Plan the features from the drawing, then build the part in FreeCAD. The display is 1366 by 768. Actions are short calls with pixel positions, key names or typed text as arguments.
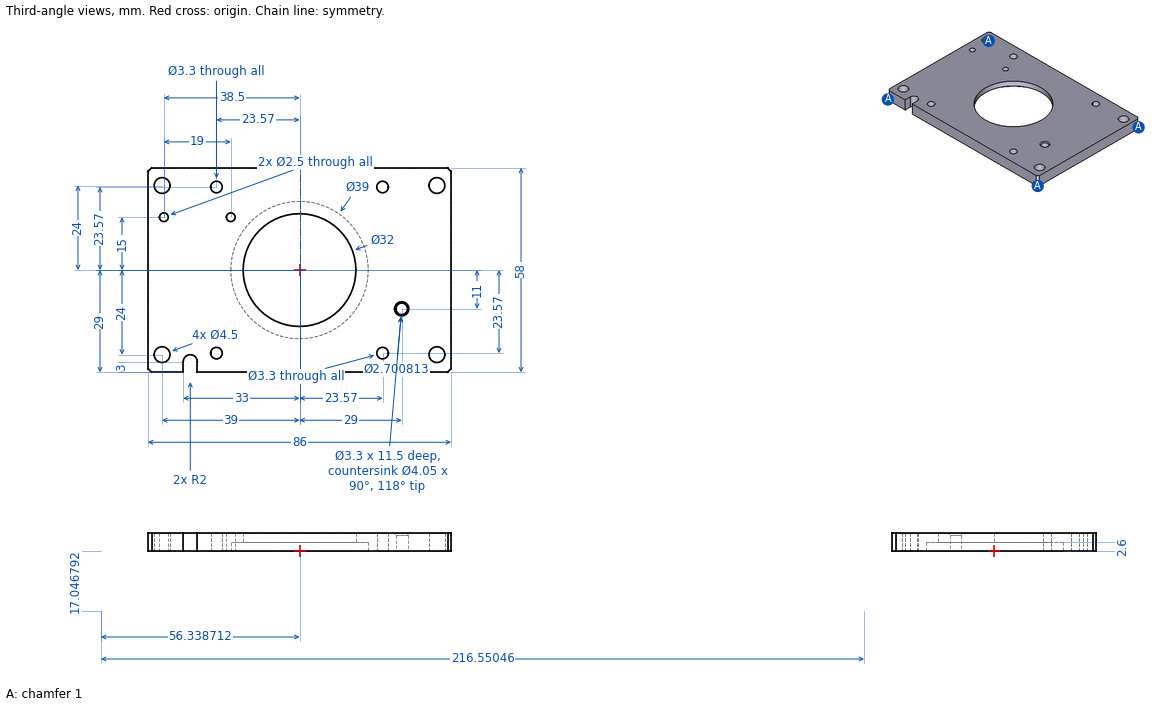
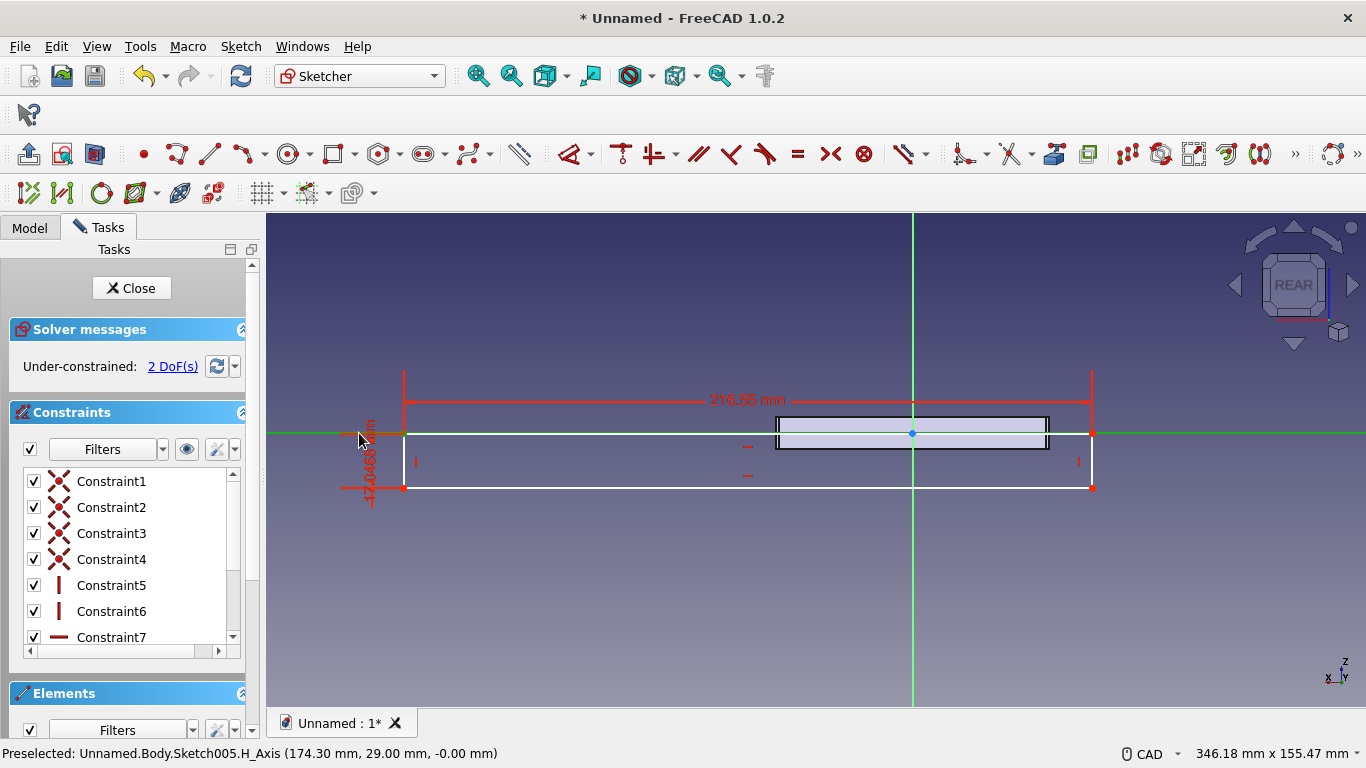
click(621, 154)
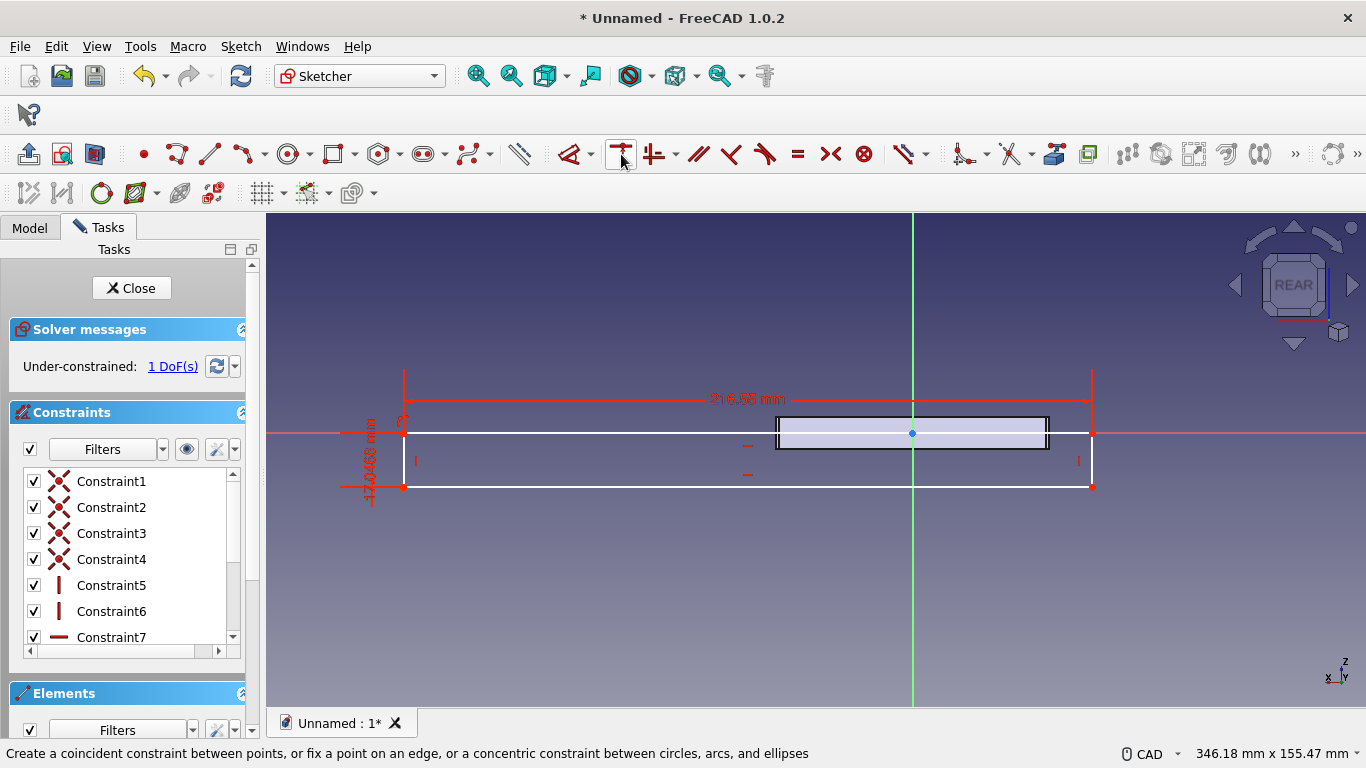
key(d)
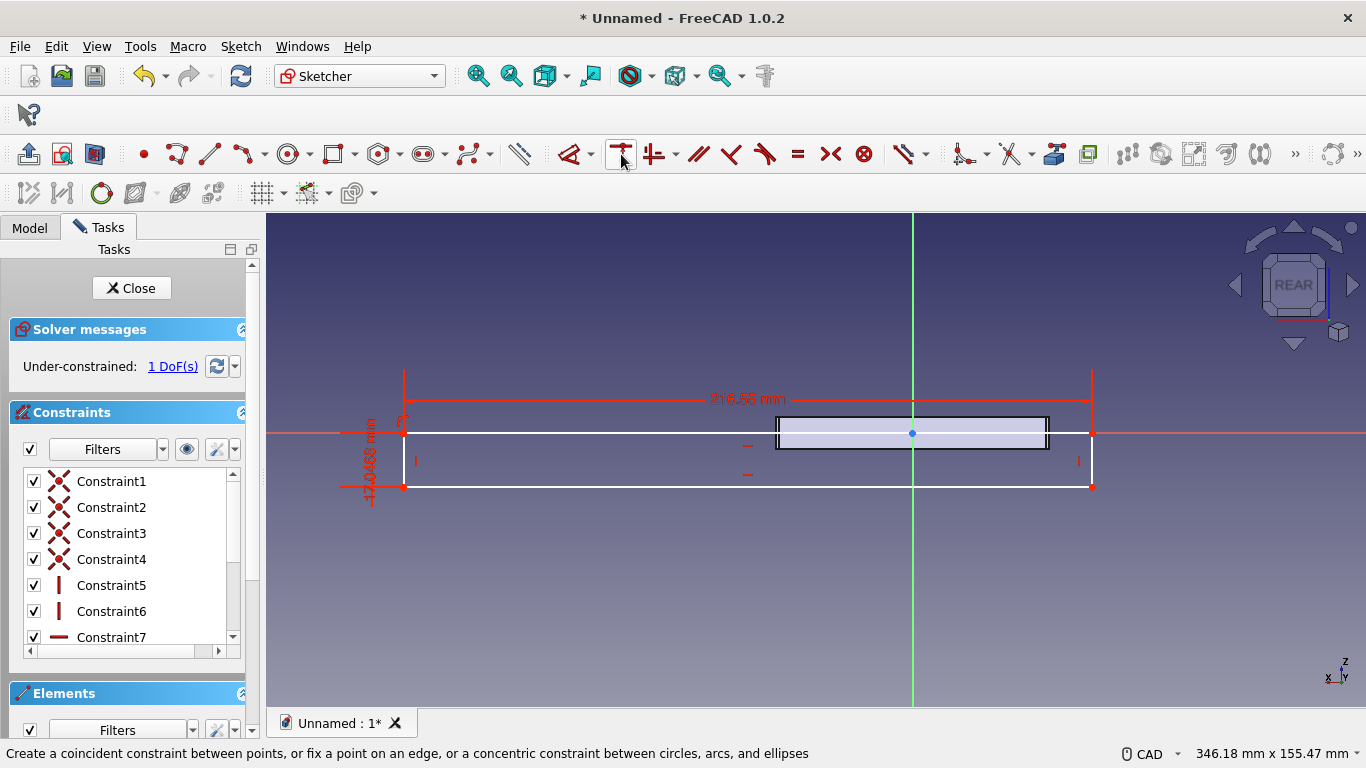
click(1092, 487)
click(1002, 399)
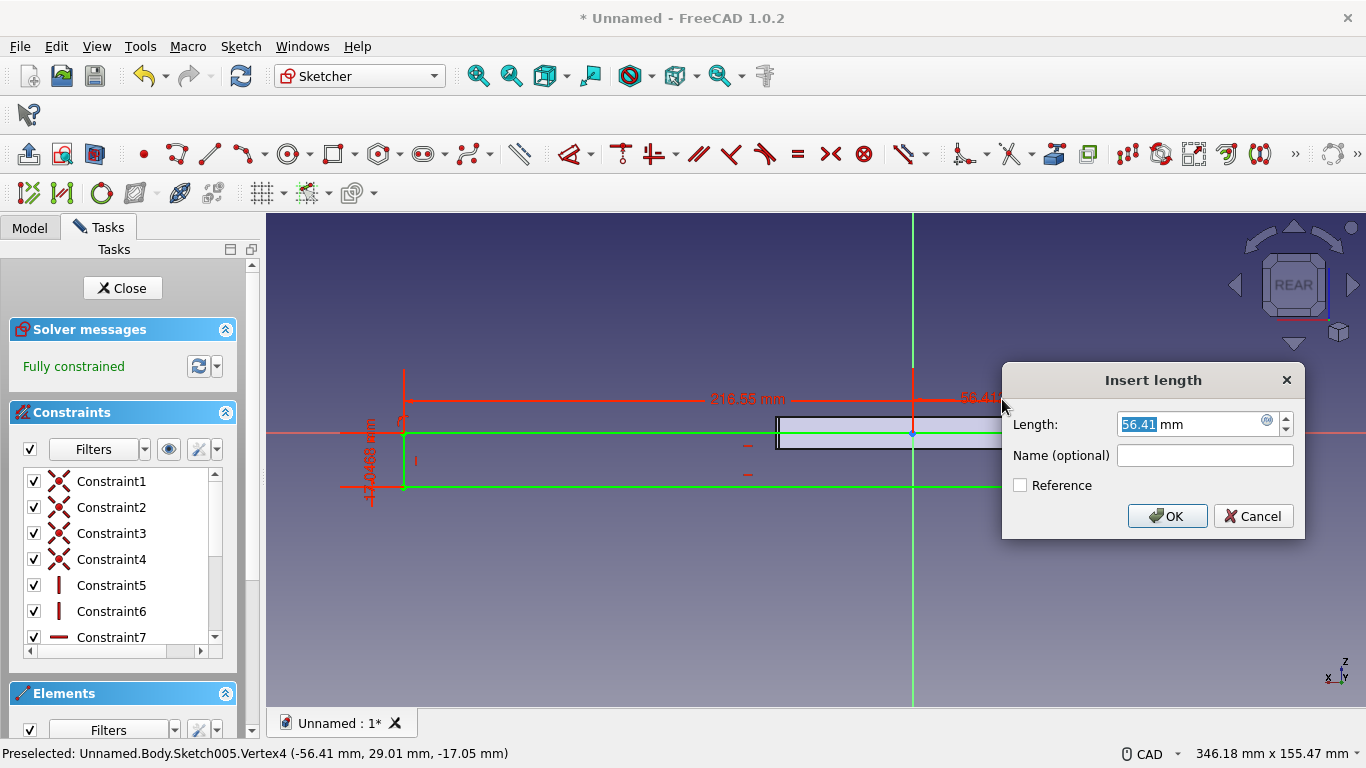
text(56.338712)
key(Return)
key(Escape)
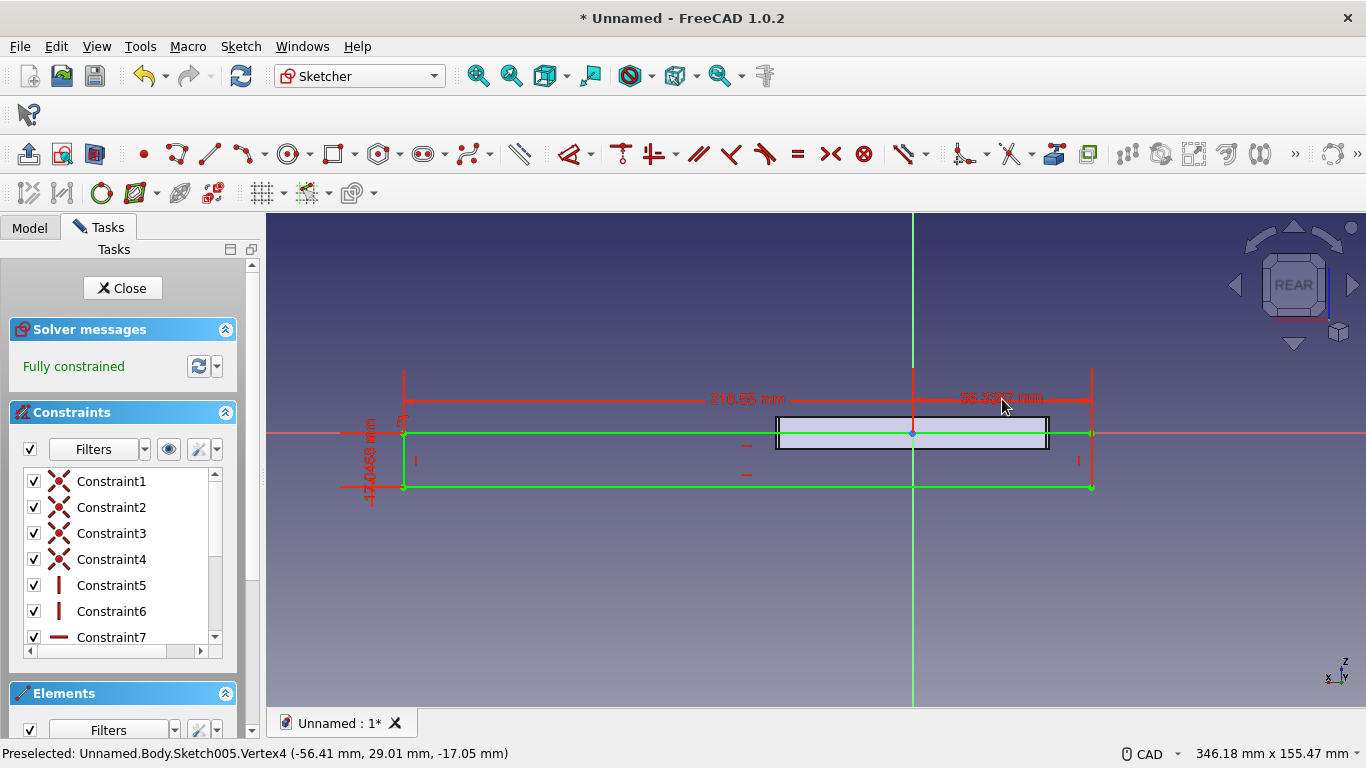
click(123, 288)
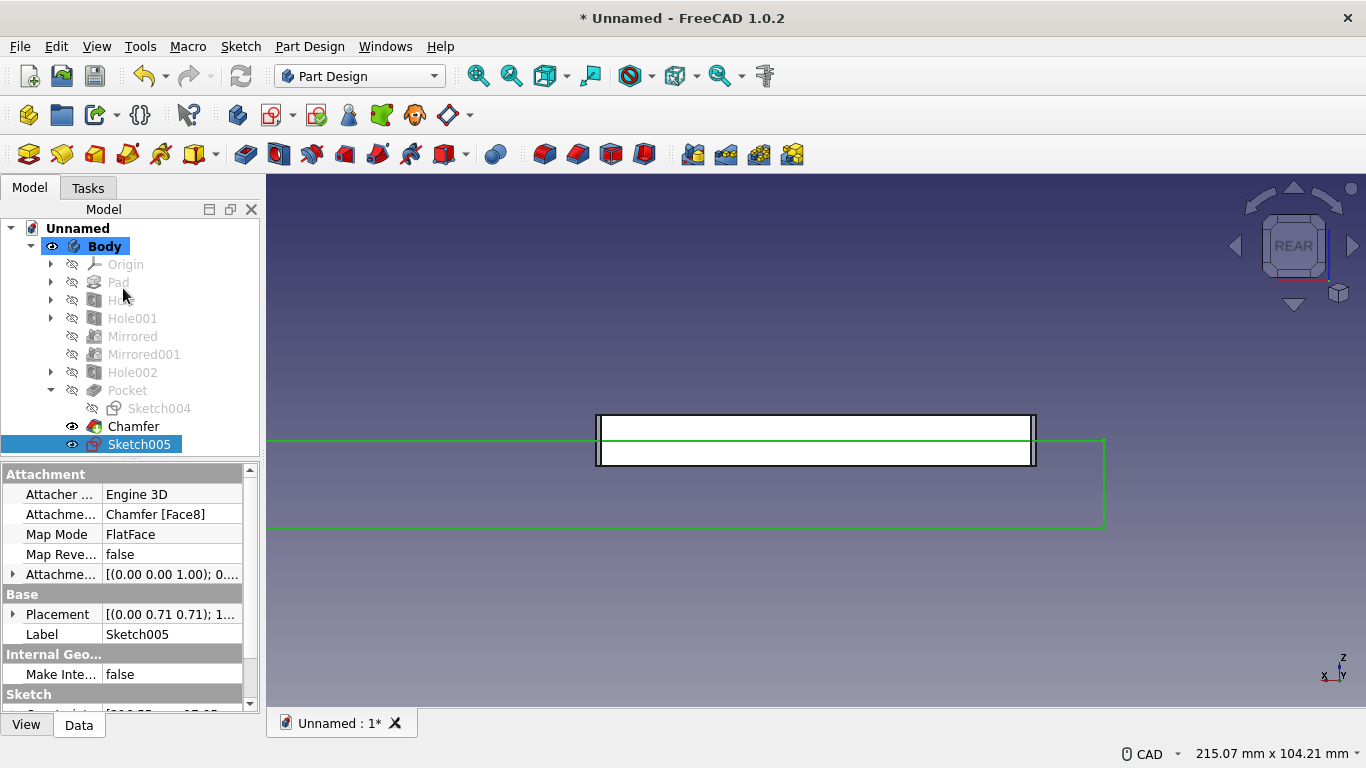
click(246, 154)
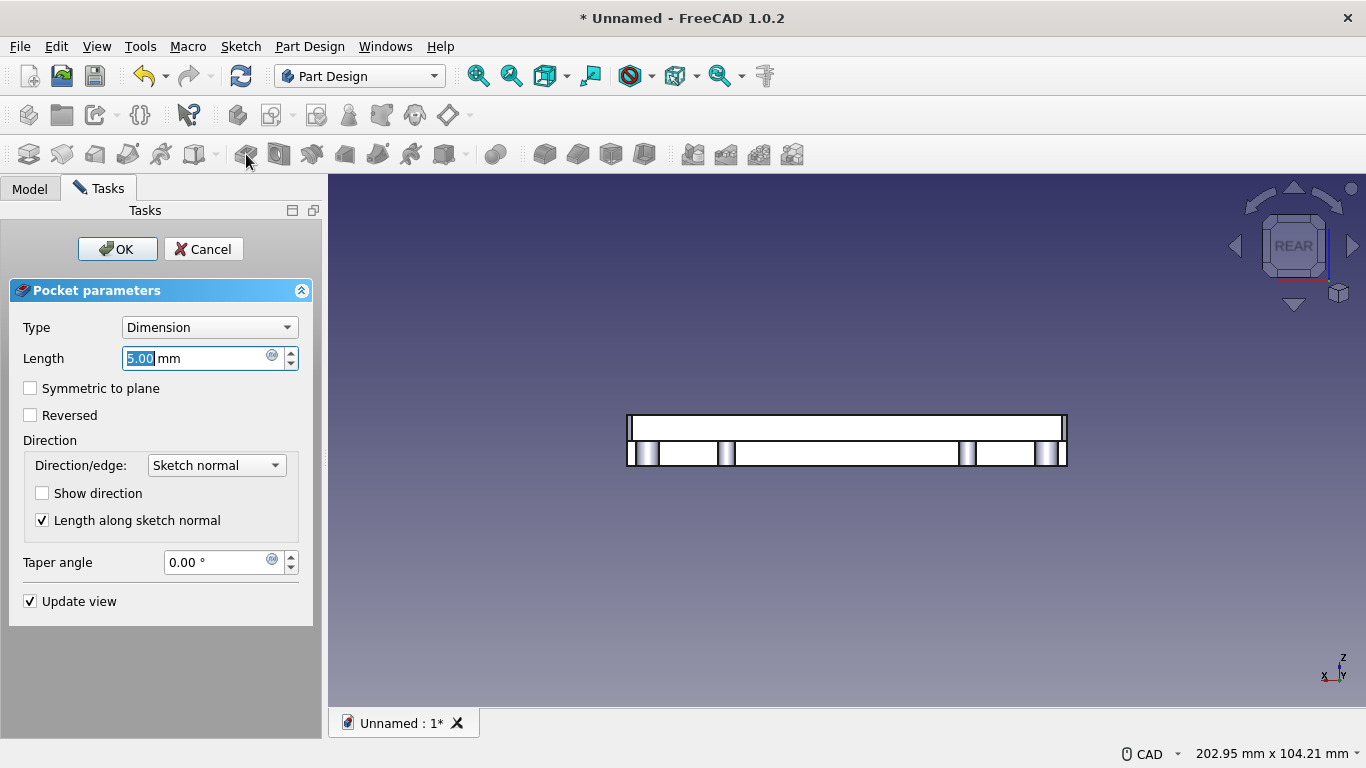
click(210, 328)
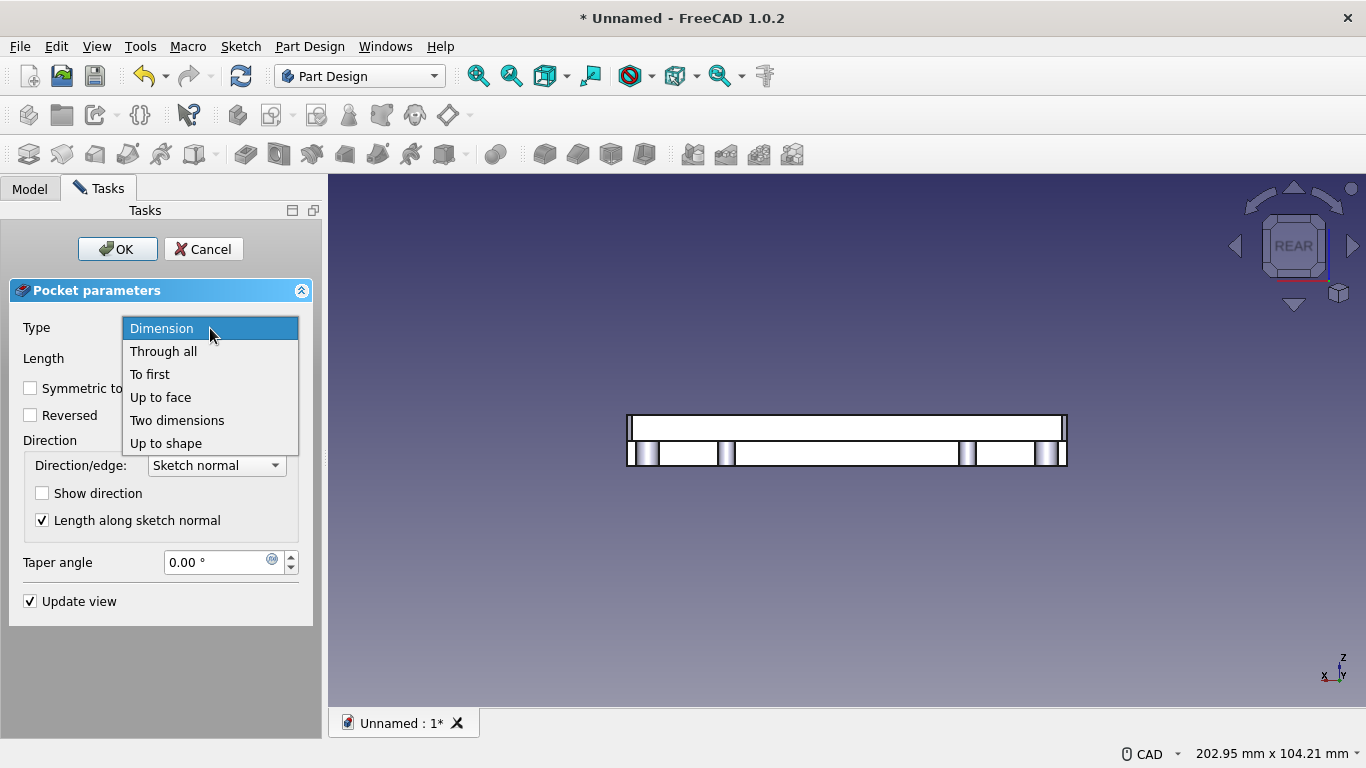
click(208, 352)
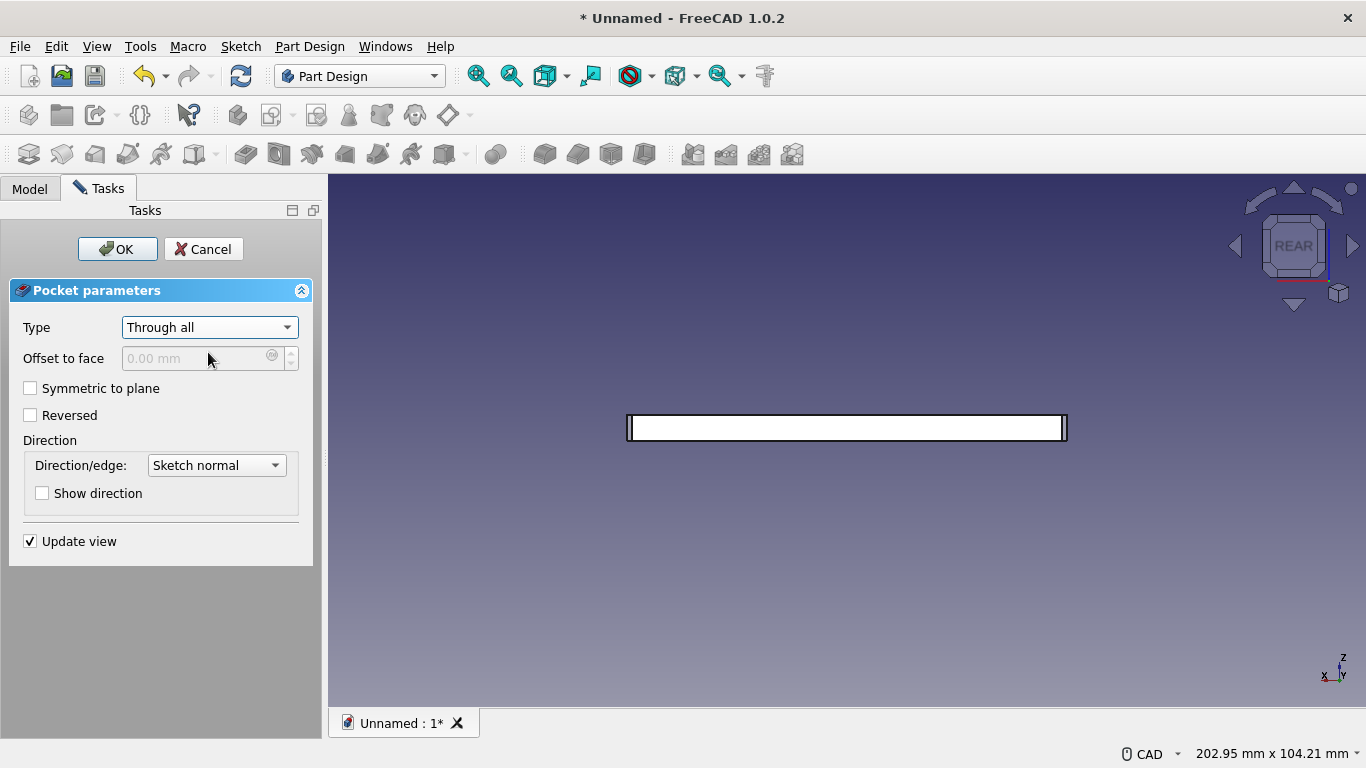
click(118, 249)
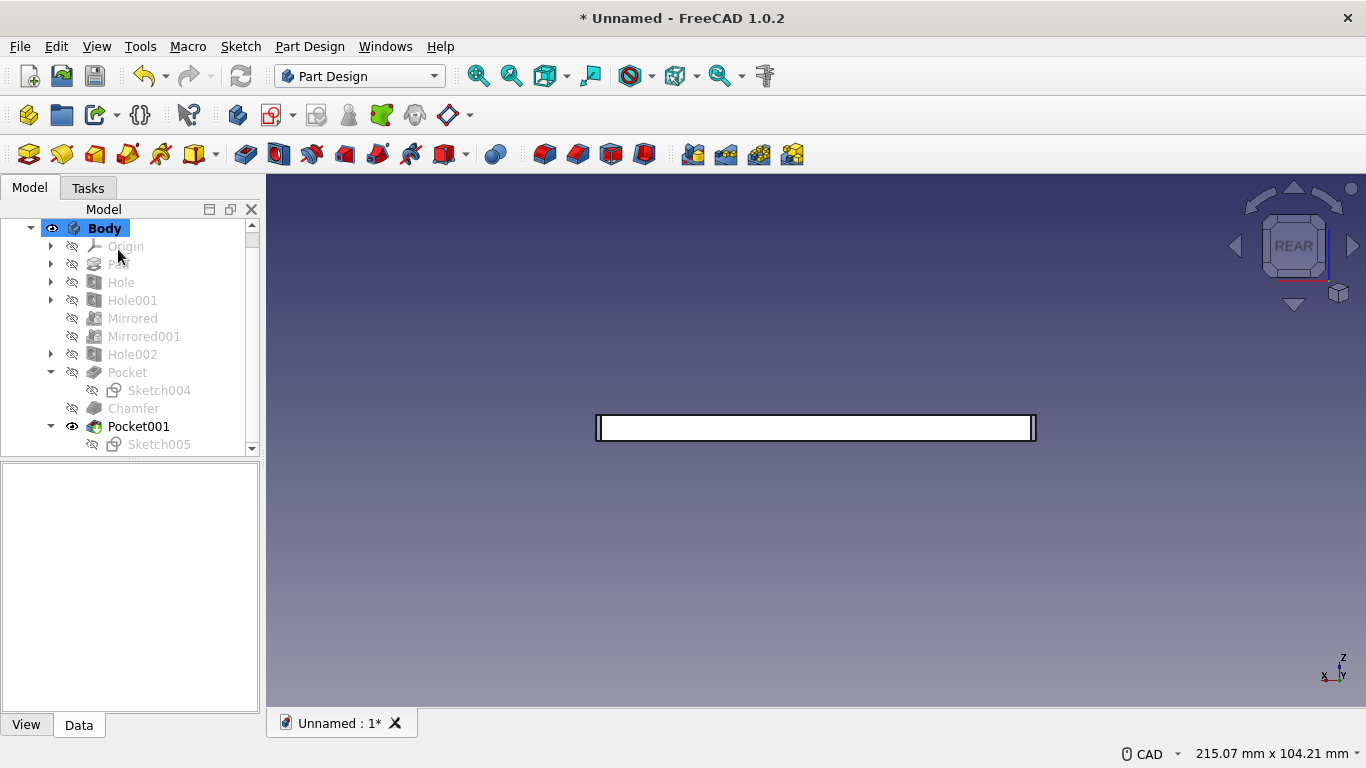
key(v)
key(f)